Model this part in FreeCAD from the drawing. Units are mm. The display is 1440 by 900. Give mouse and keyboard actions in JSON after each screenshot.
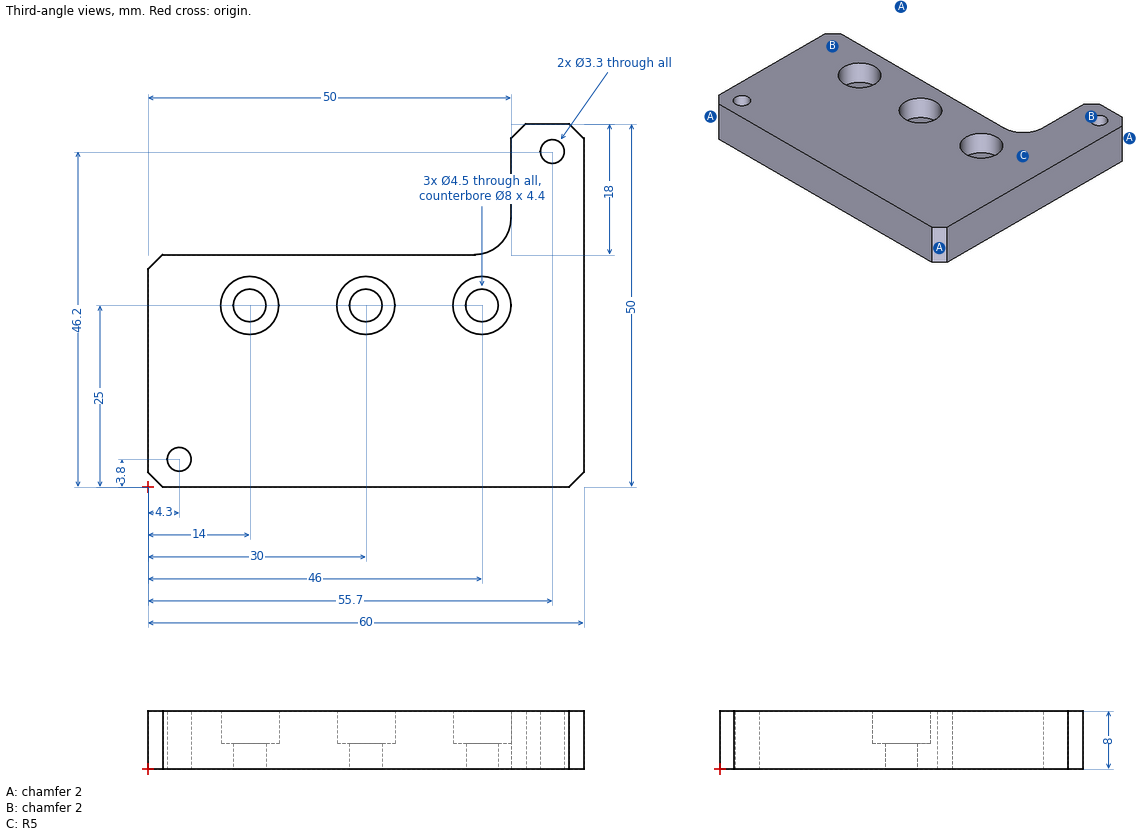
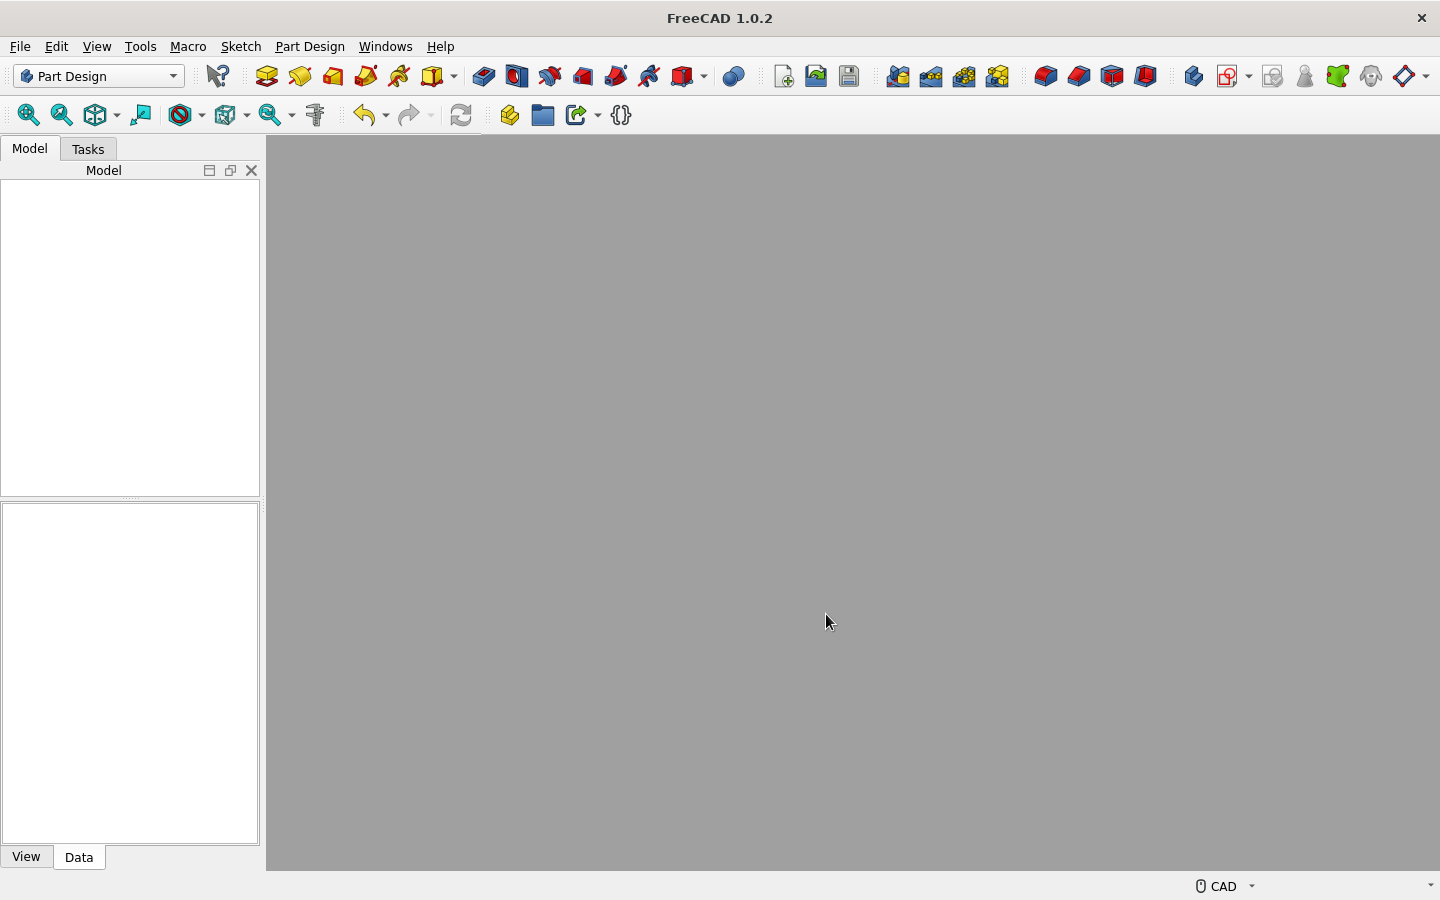
{"action": "left_click", "coordinate": [783, 76]}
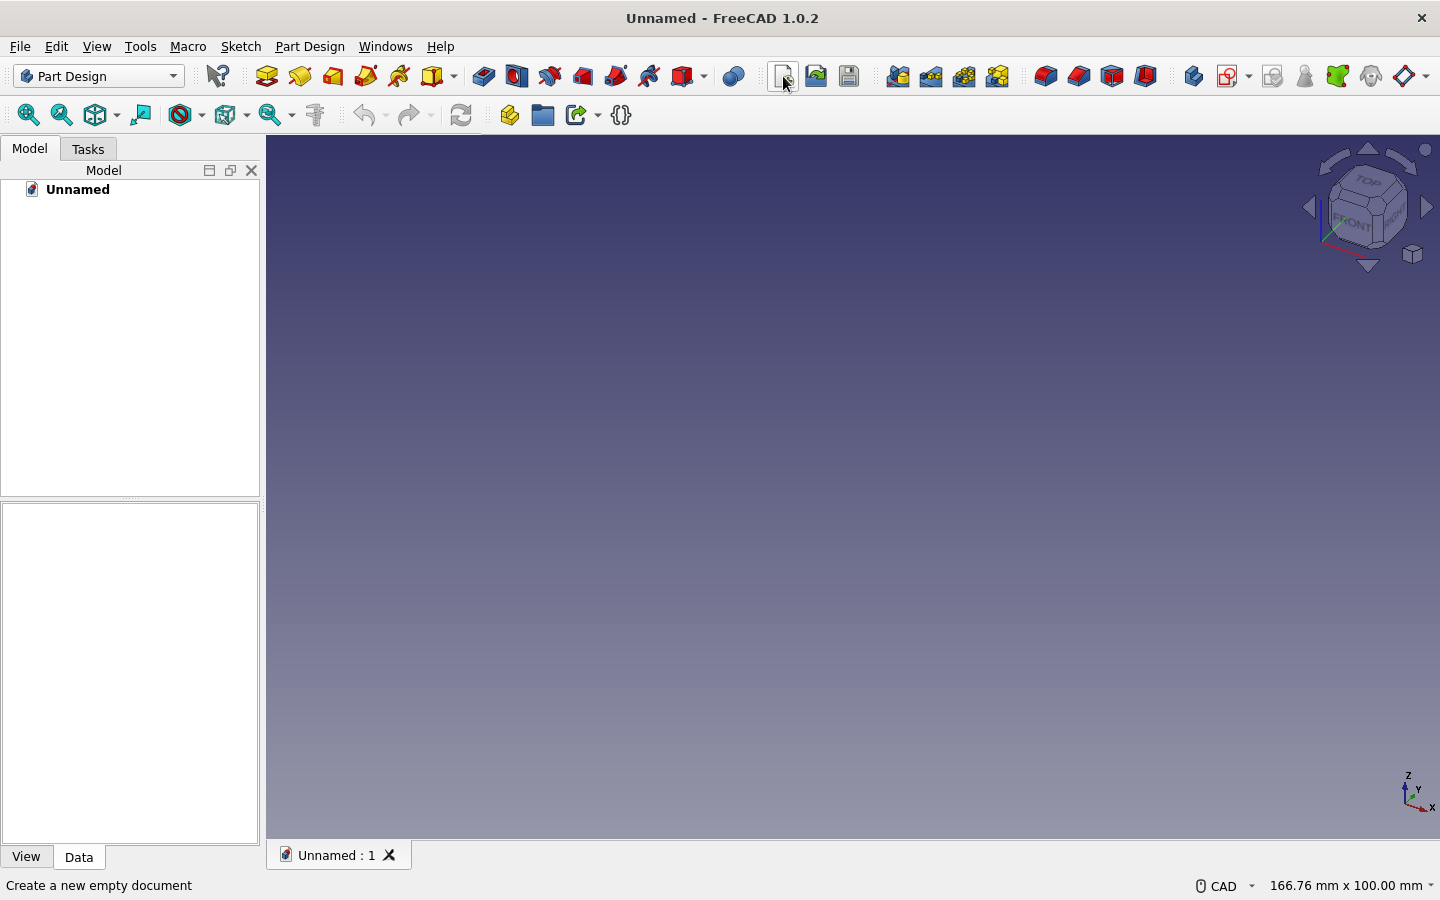
{"action": "left_click", "coordinate": [1226, 76]}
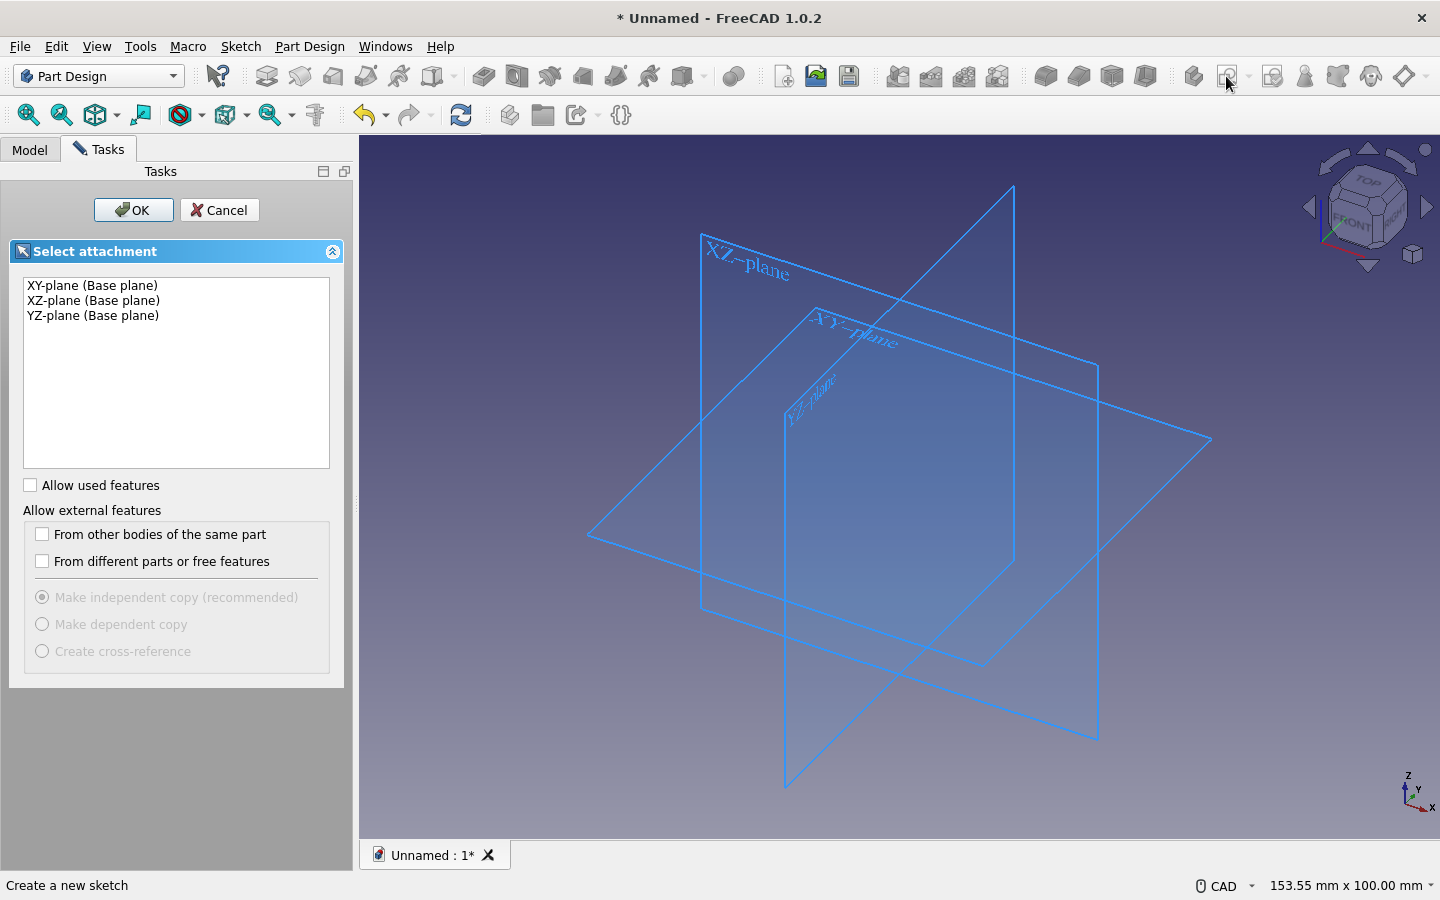
{"action": "left_click", "coordinate": [84, 286]}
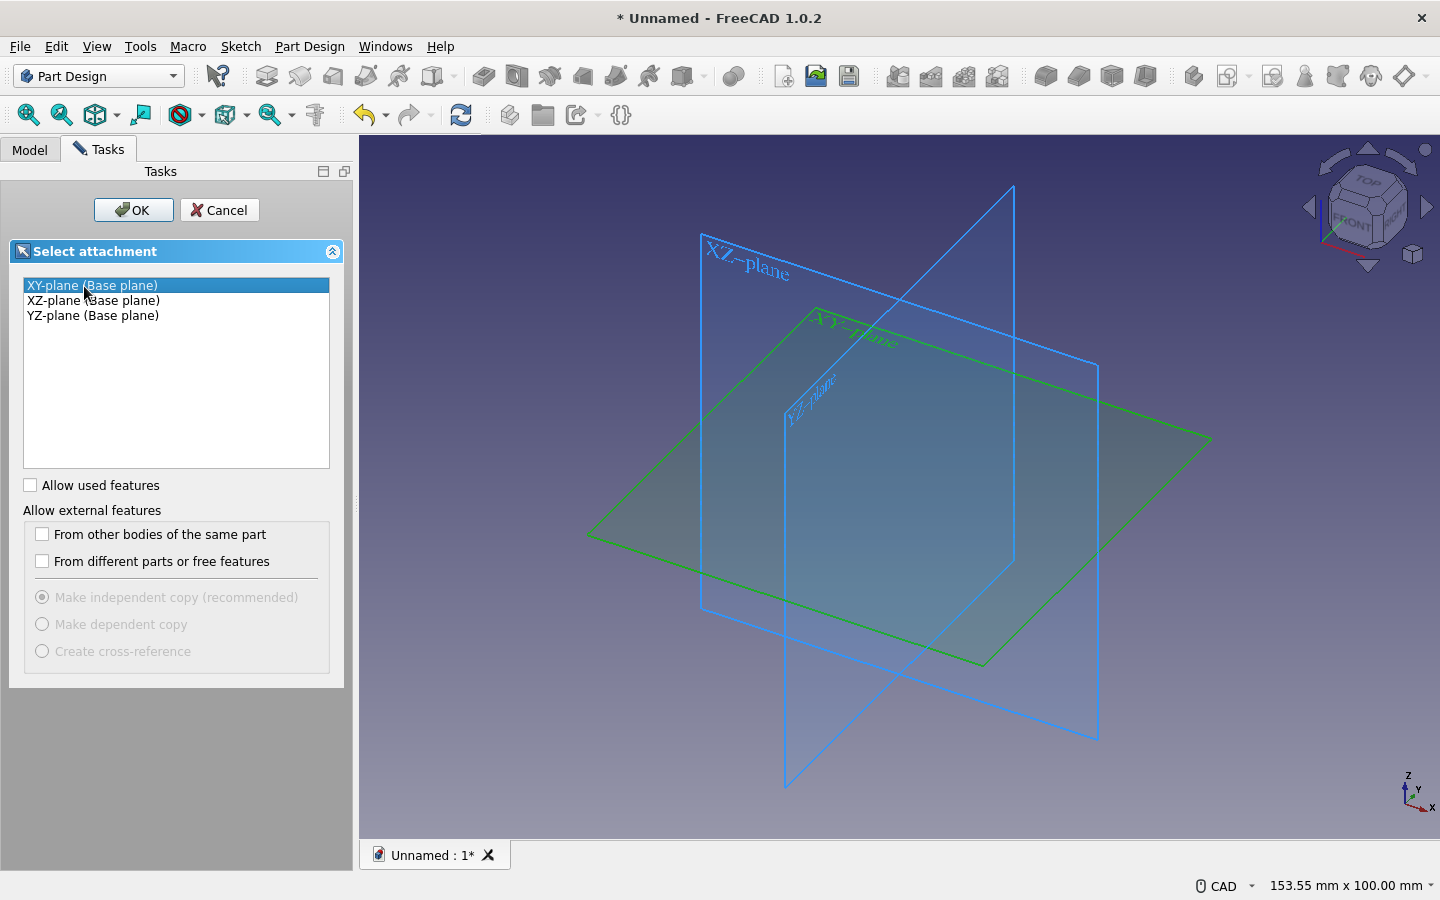
{"action": "left_click", "coordinate": [134, 210]}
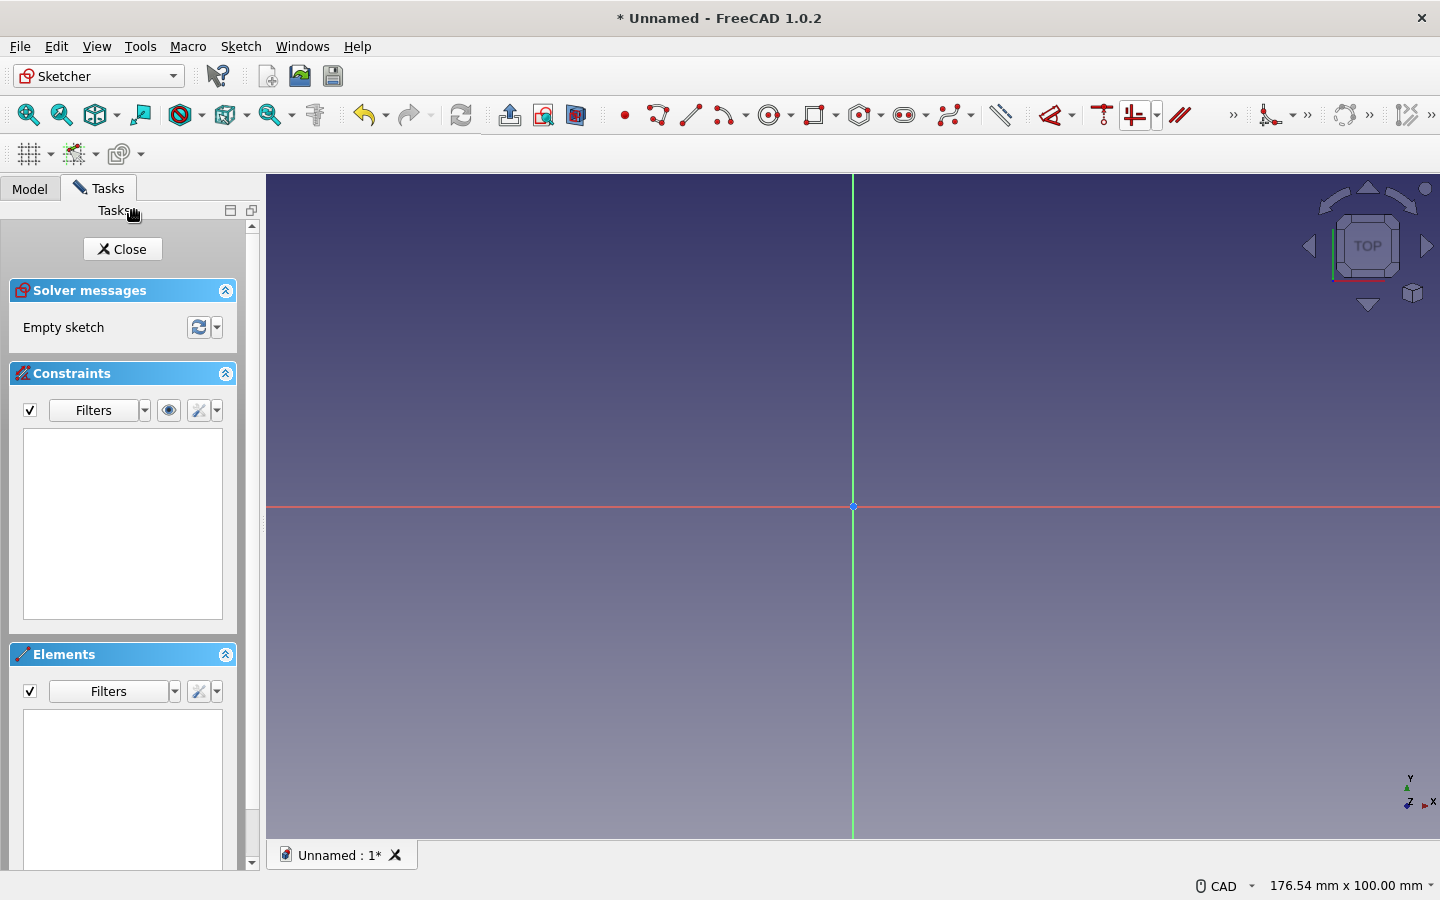
{"action": "scroll", "coordinate": [294, 811], "scroll_direction": "down", "scroll_amount": 1}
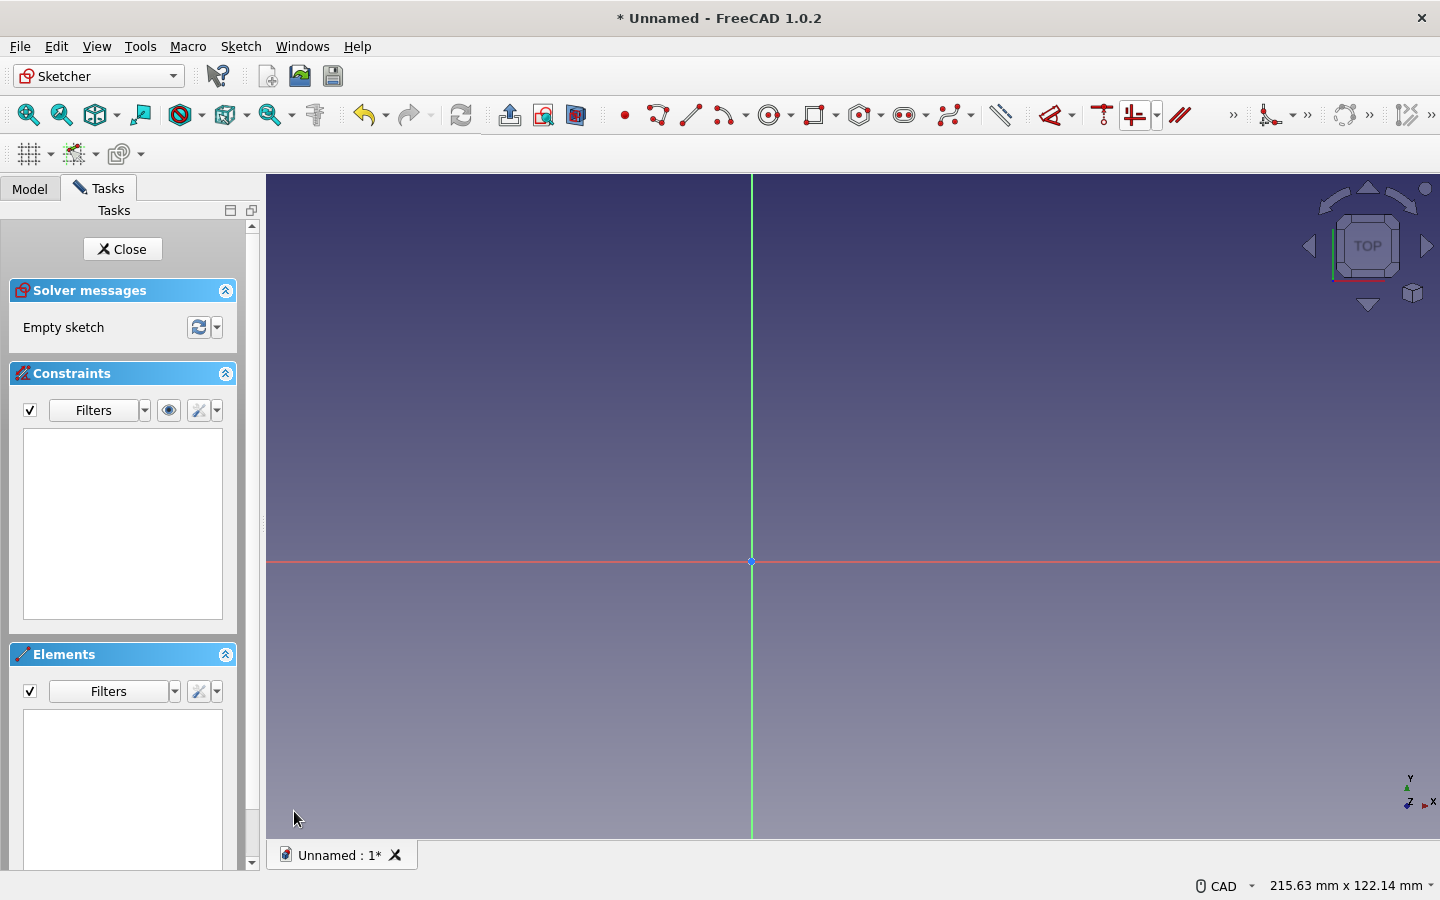
{"action": "scroll", "coordinate": [1180, 262], "scroll_direction": "up", "scroll_amount": 2}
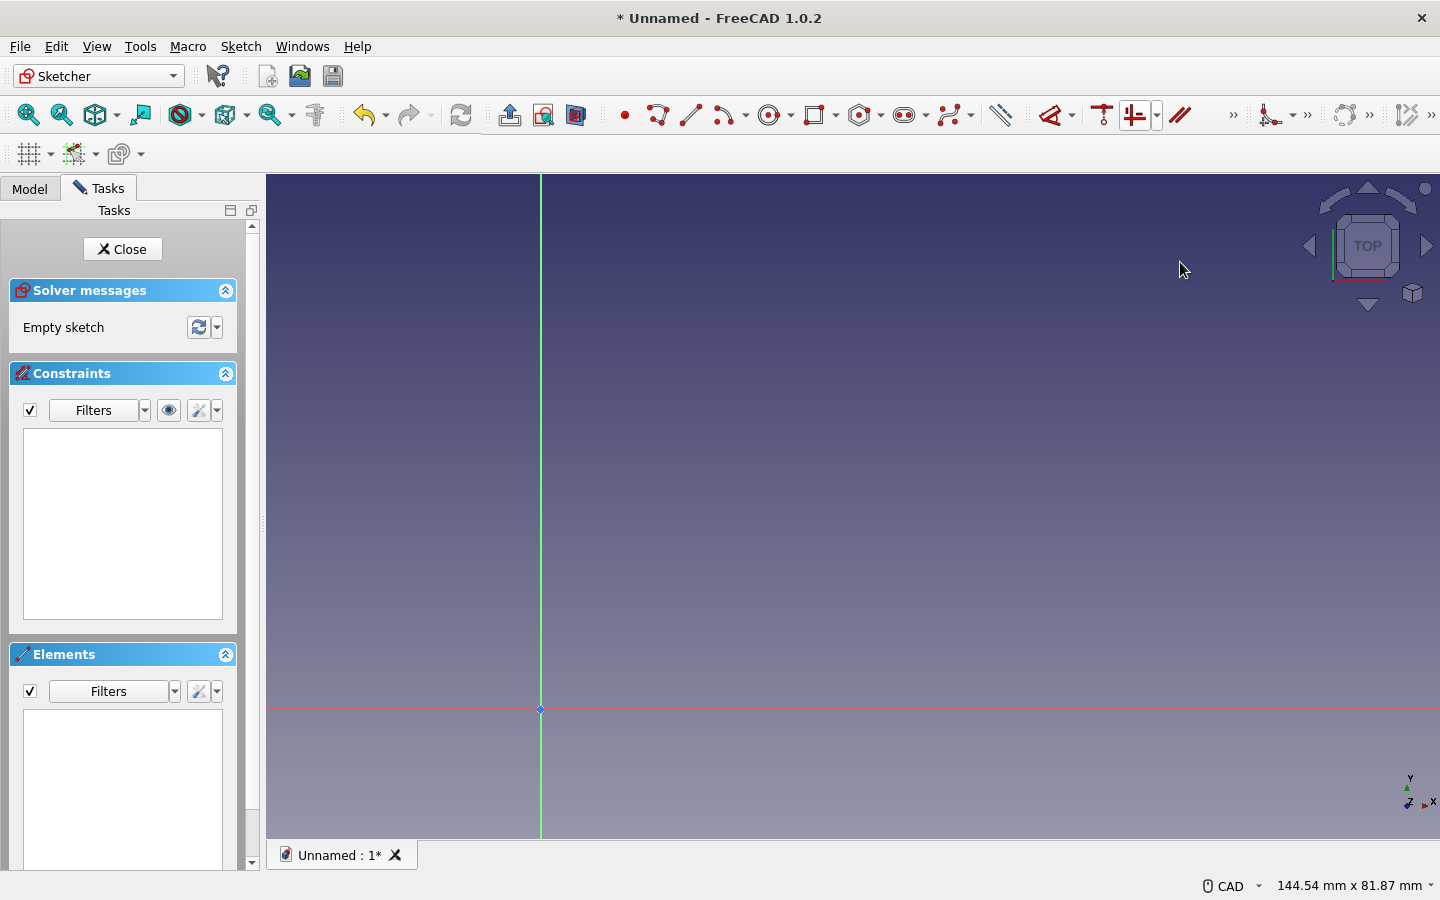
{"action": "left_click", "coordinate": [814, 116]}